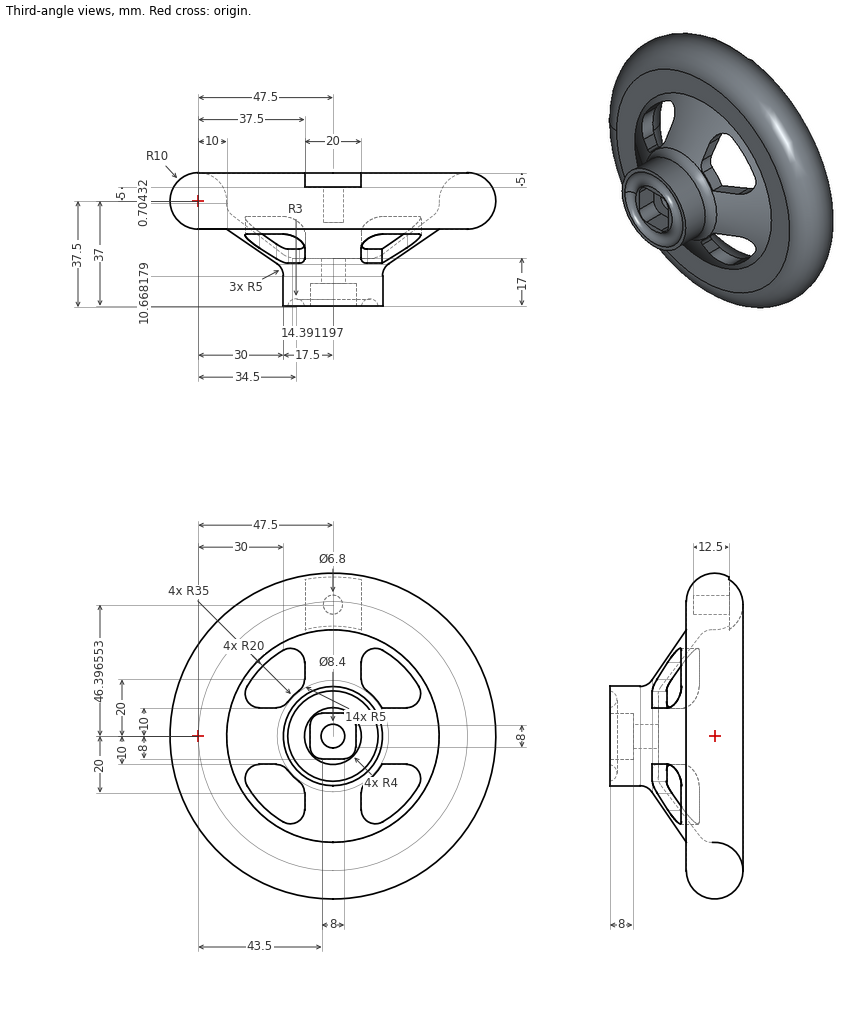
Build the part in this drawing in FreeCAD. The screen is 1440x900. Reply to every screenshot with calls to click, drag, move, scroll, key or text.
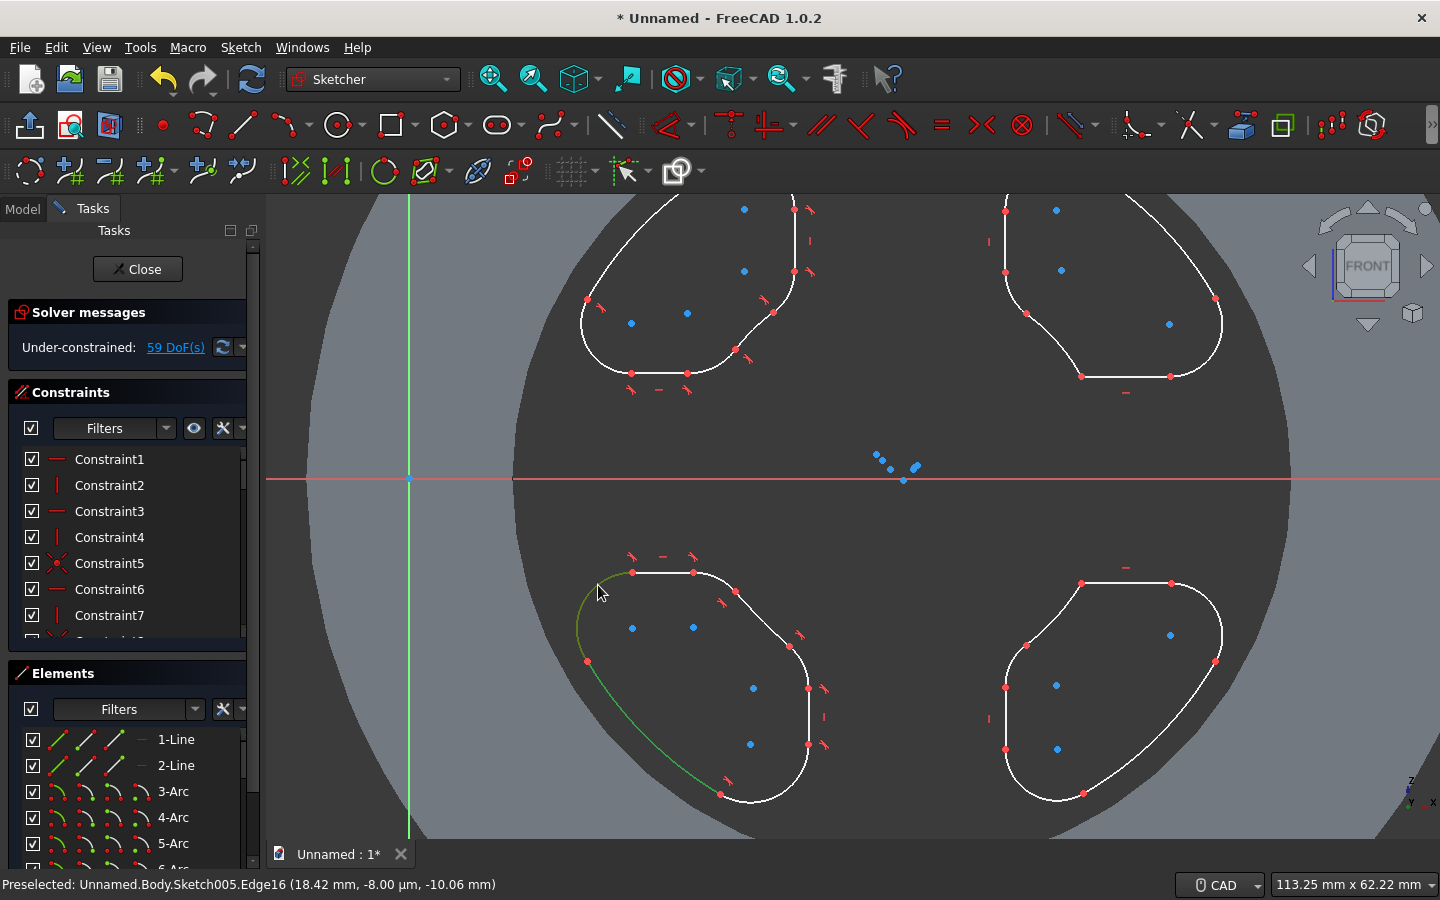
click(902, 126)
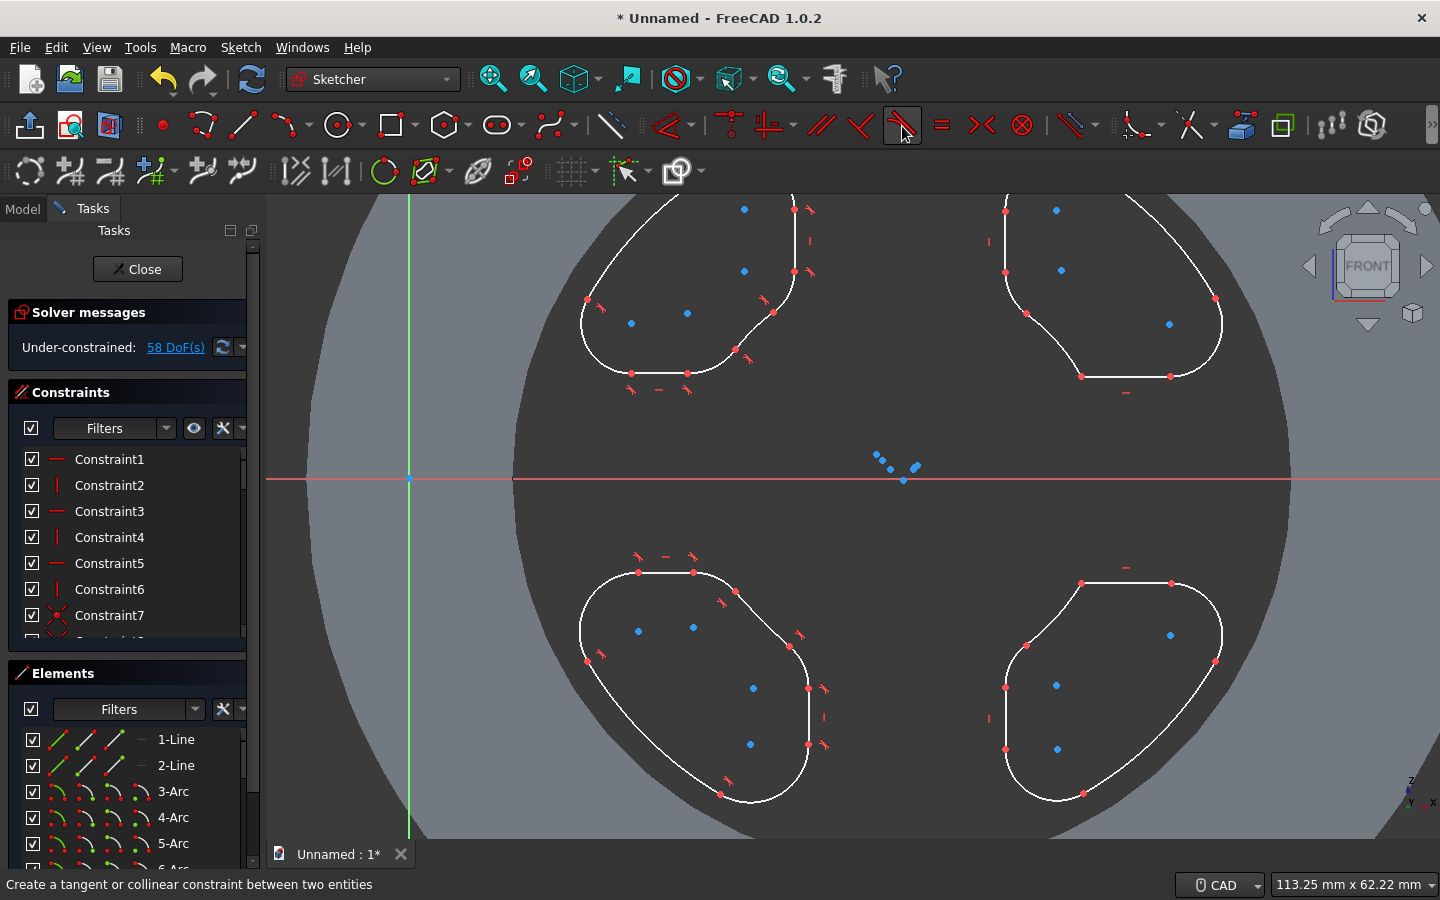
click(1108, 583)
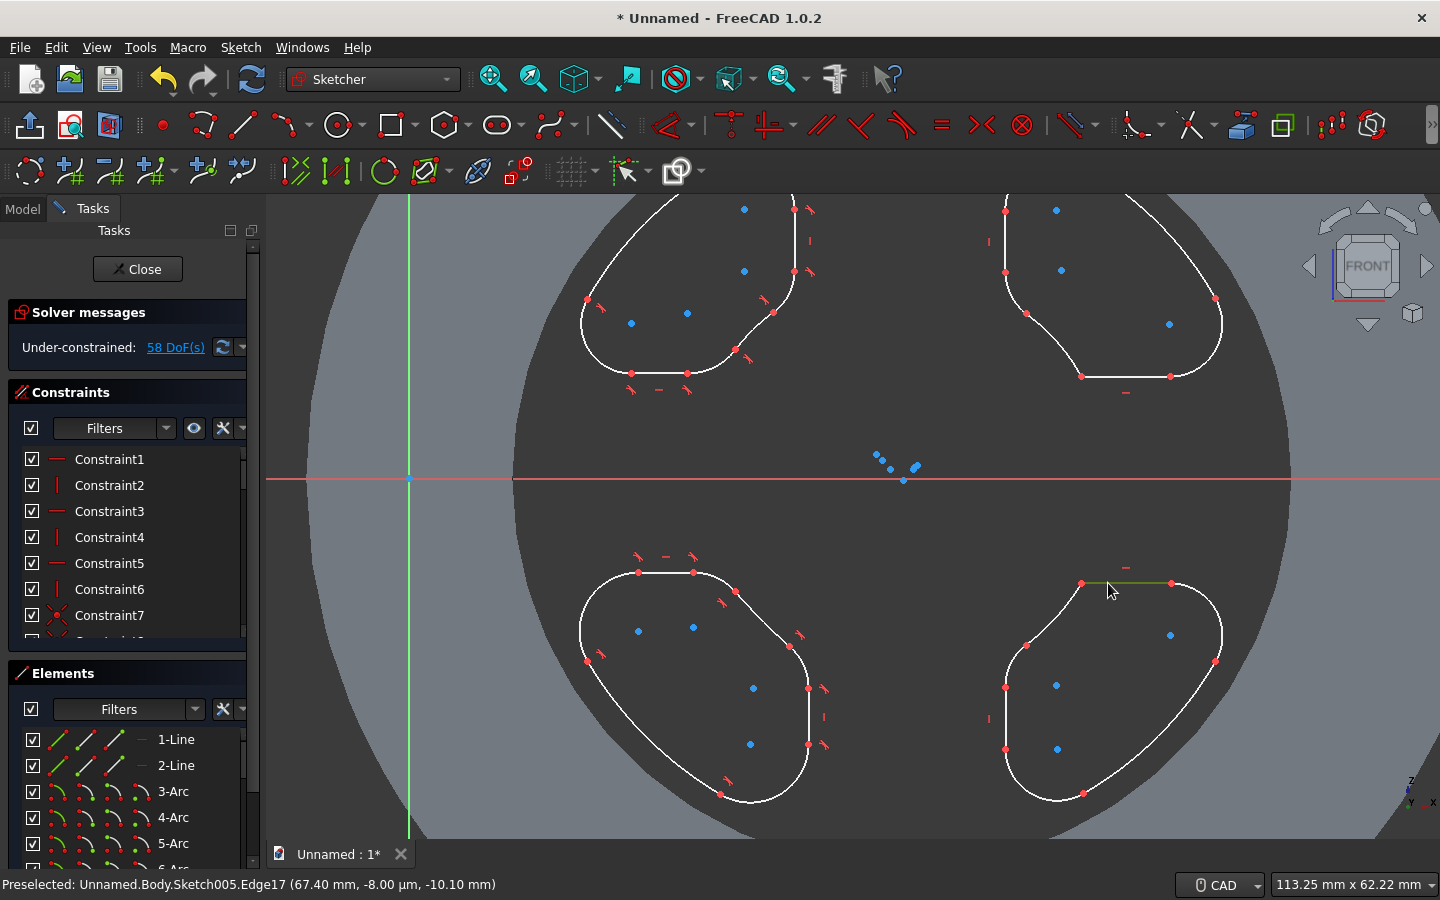
click(1222, 630)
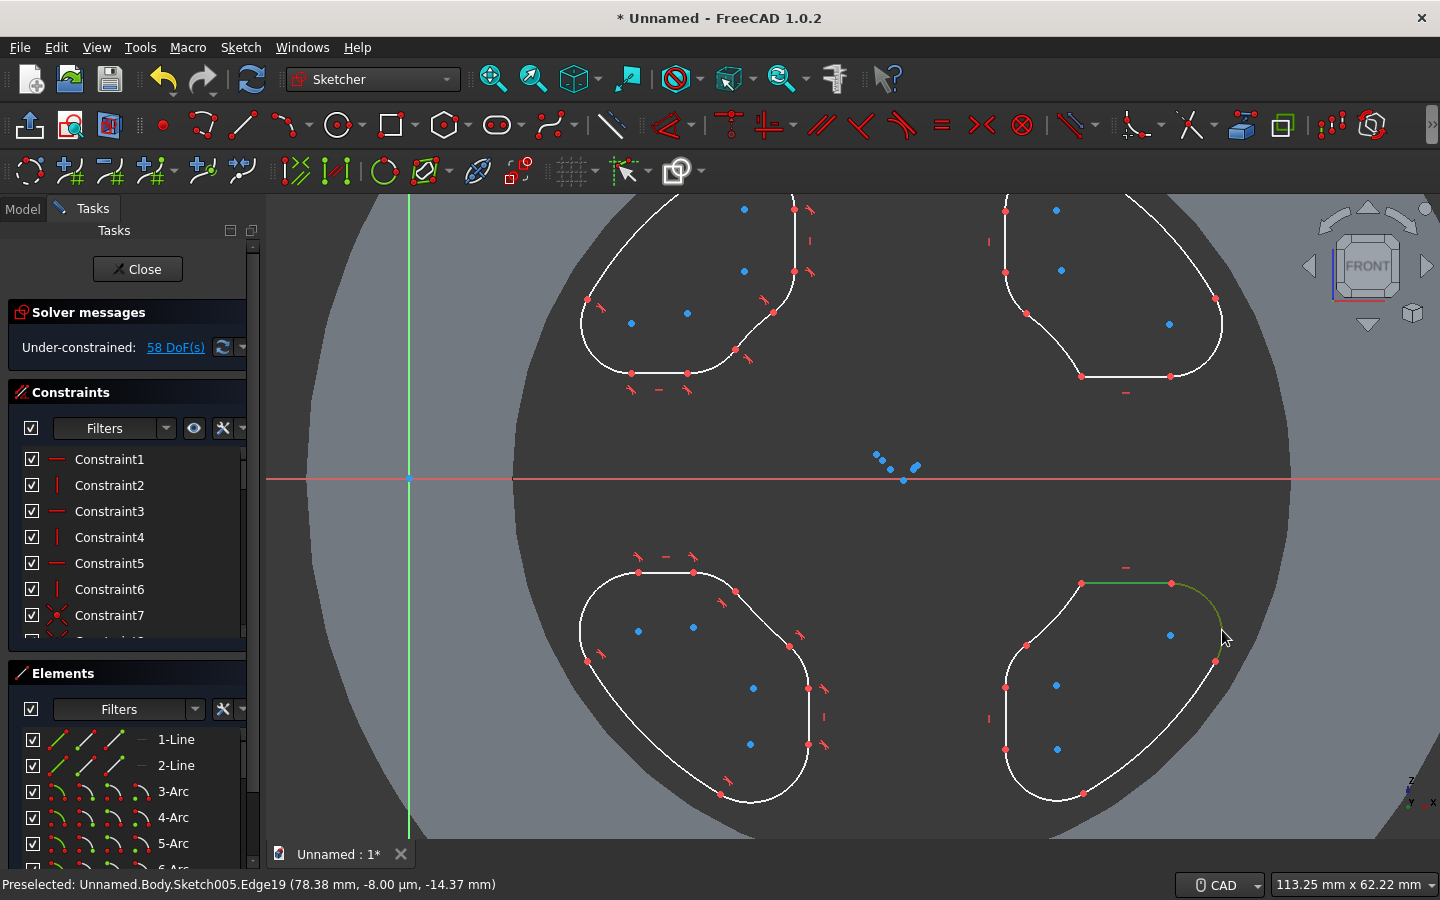
click(902, 126)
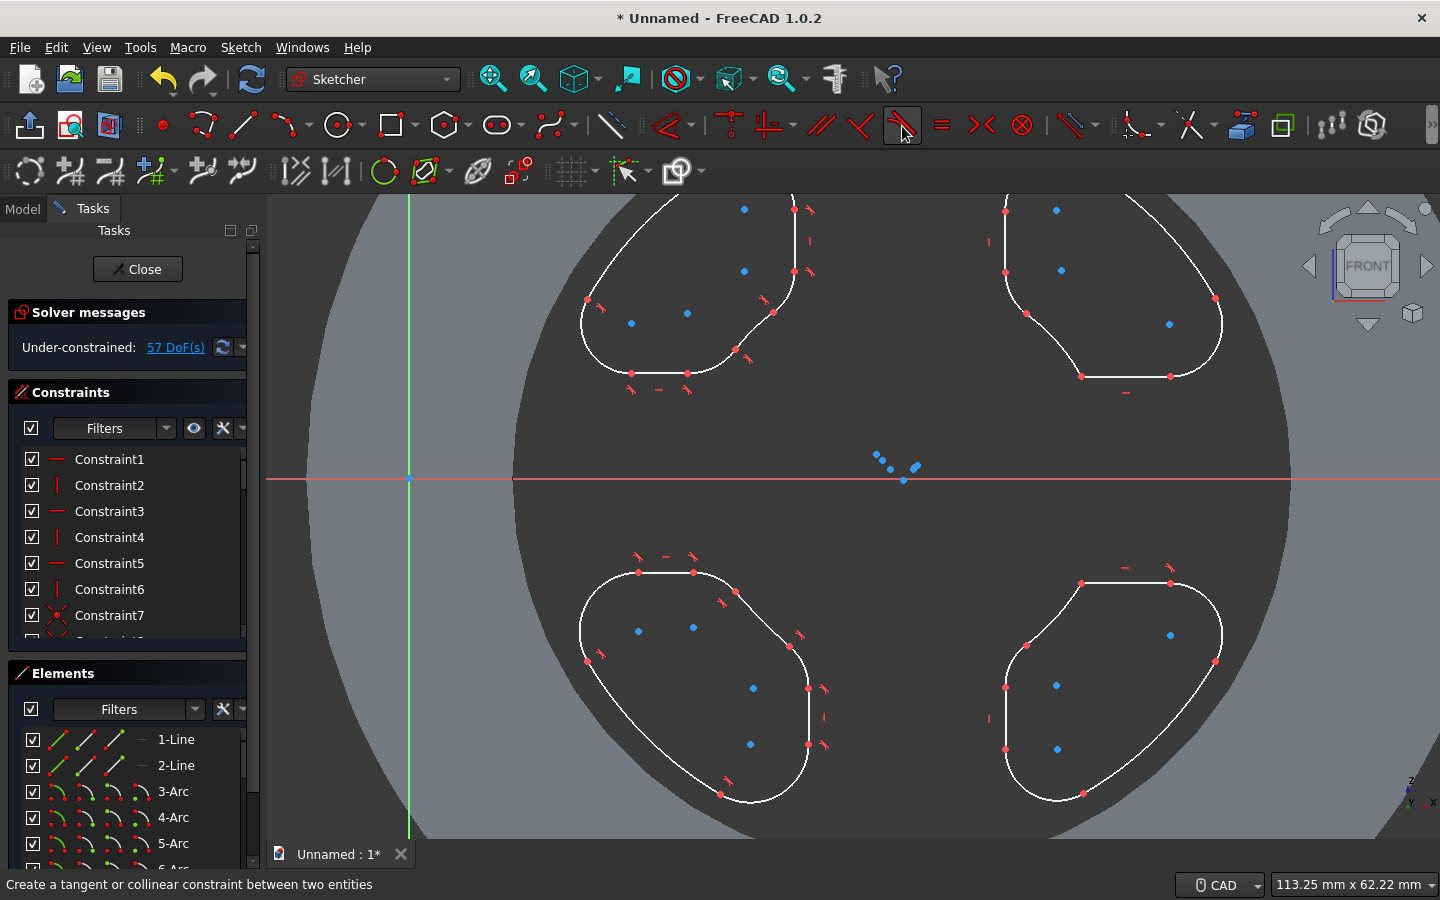
click(1006, 731)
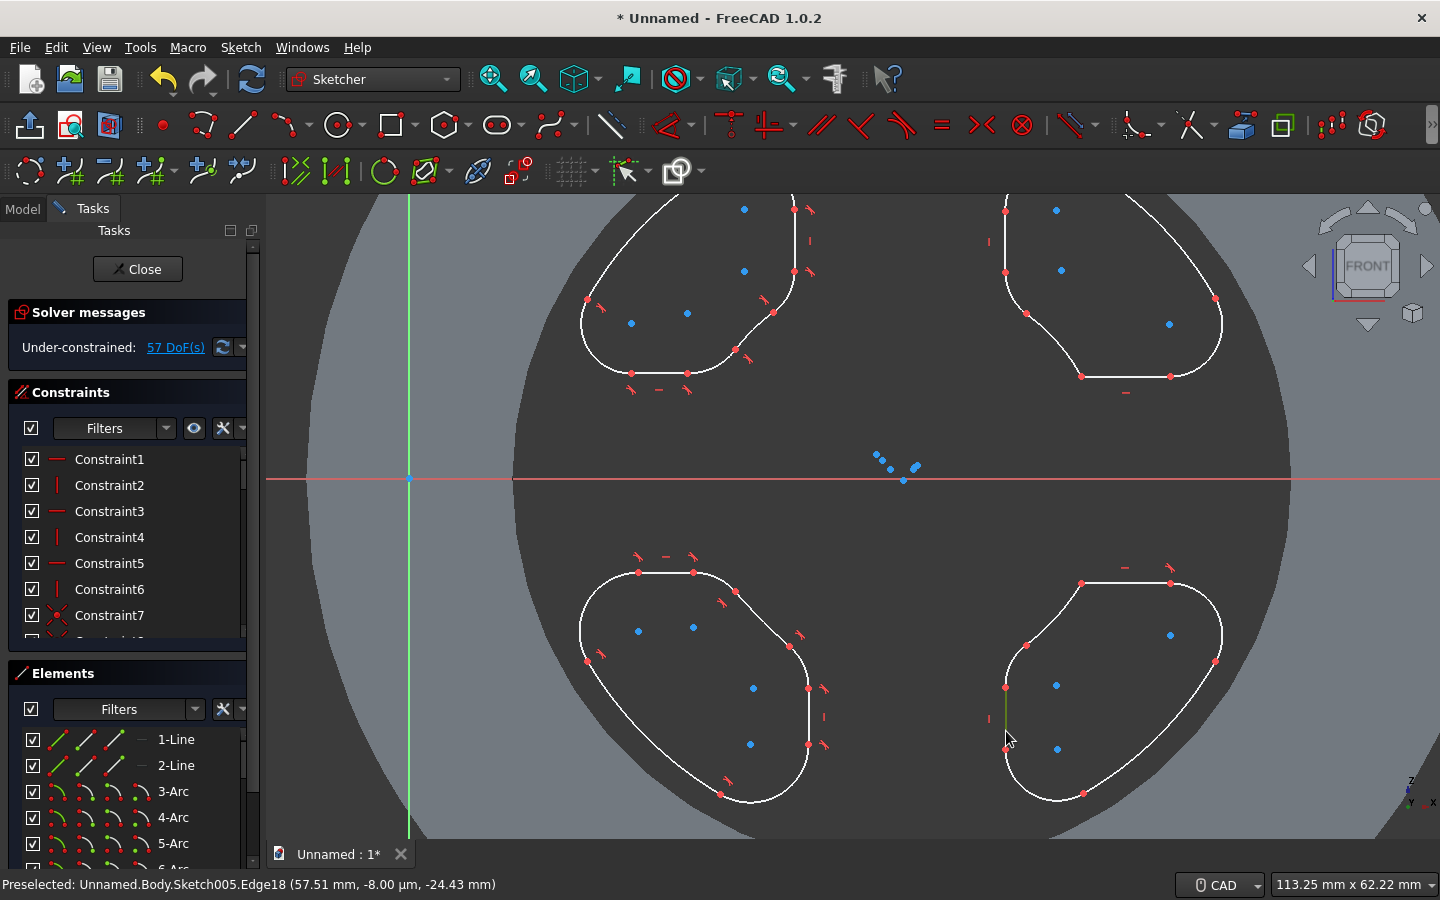
click(1015, 779)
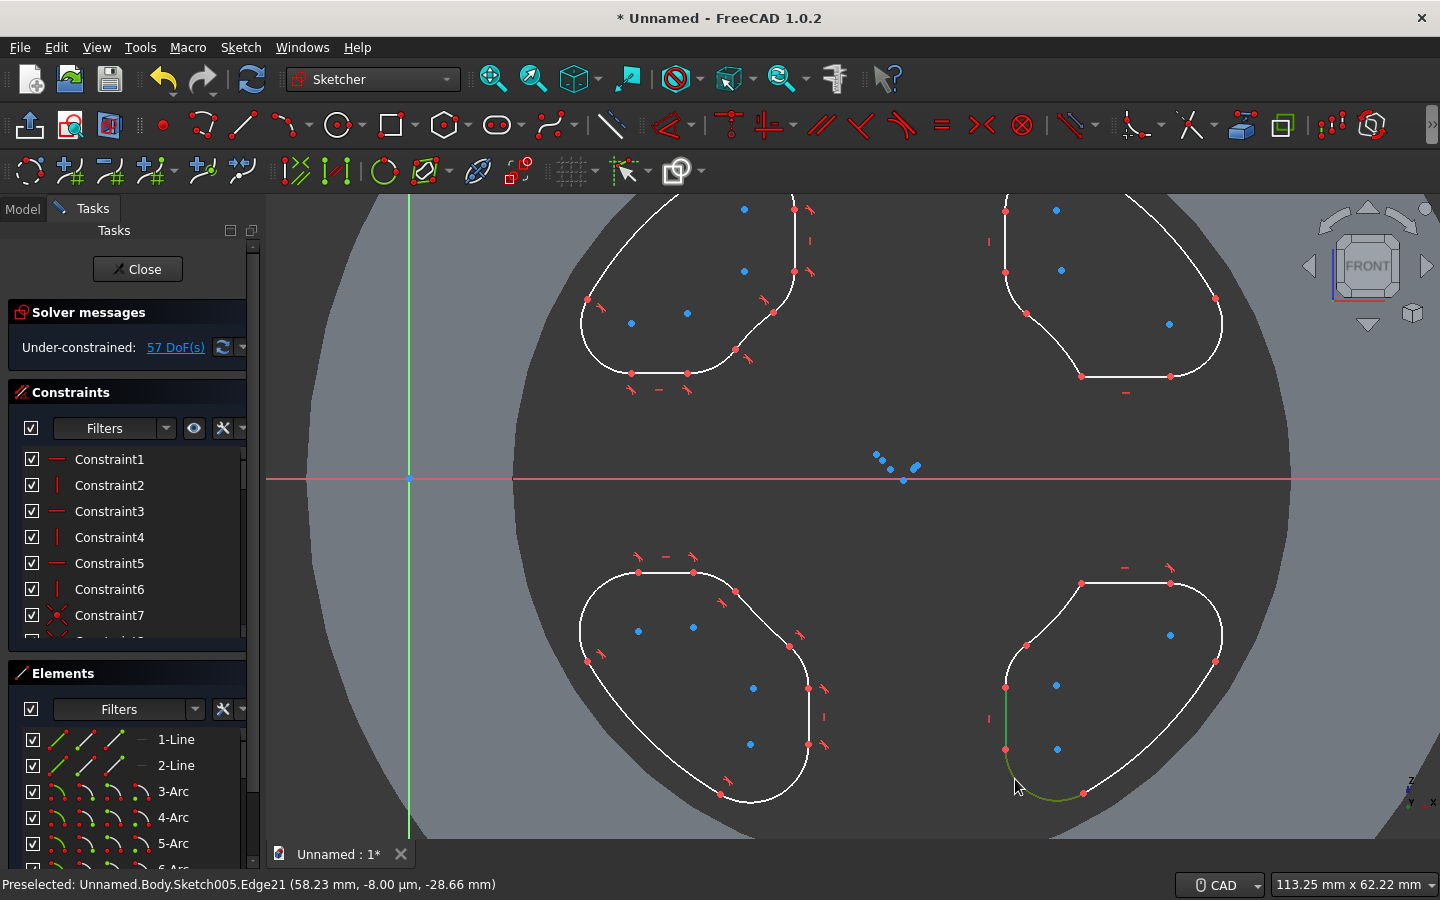
click(902, 126)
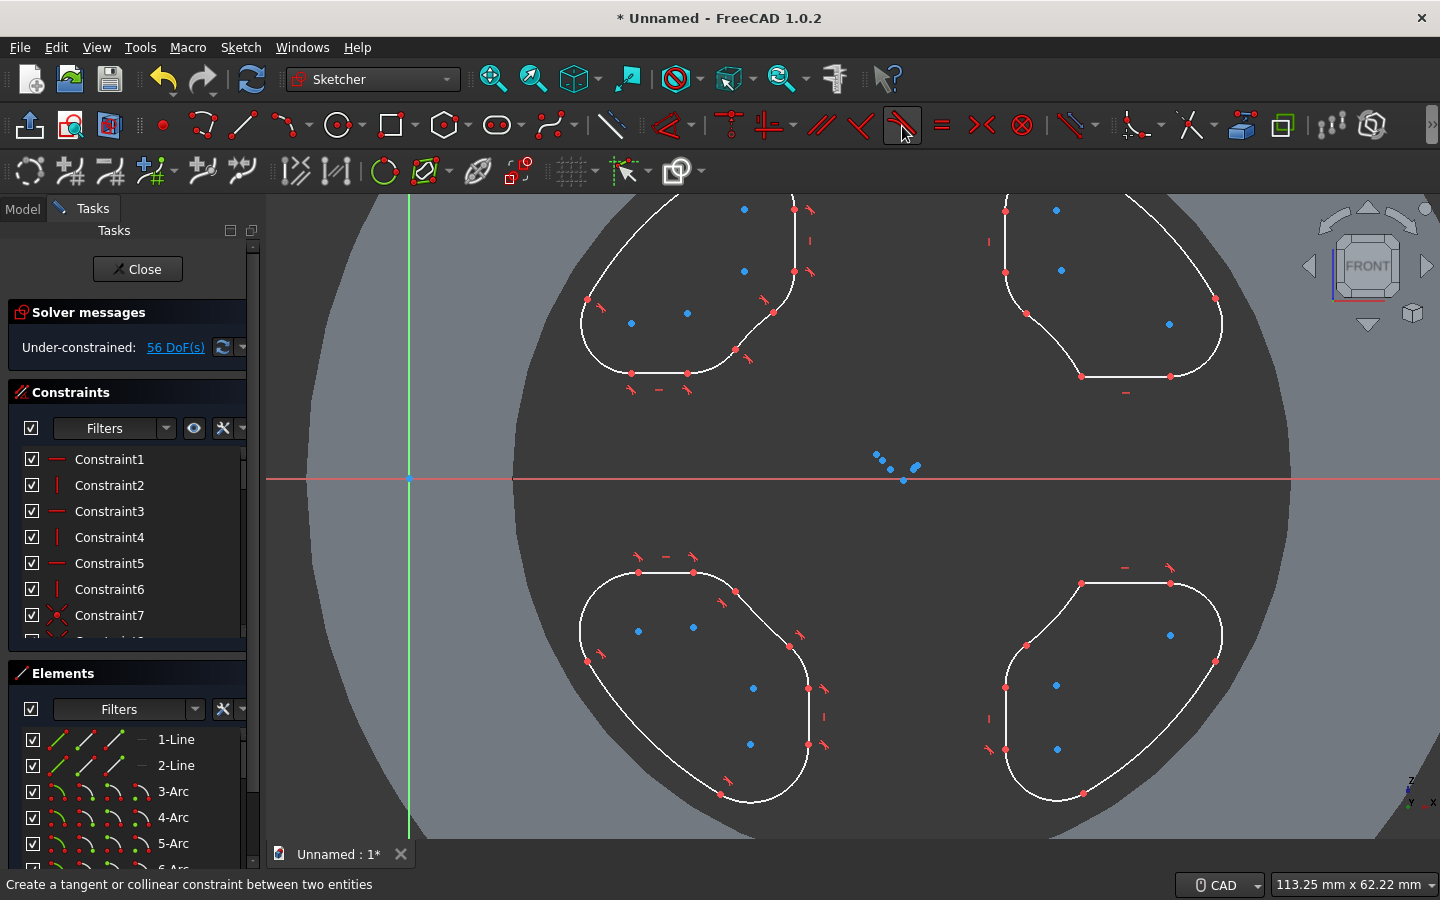
click(1006, 731)